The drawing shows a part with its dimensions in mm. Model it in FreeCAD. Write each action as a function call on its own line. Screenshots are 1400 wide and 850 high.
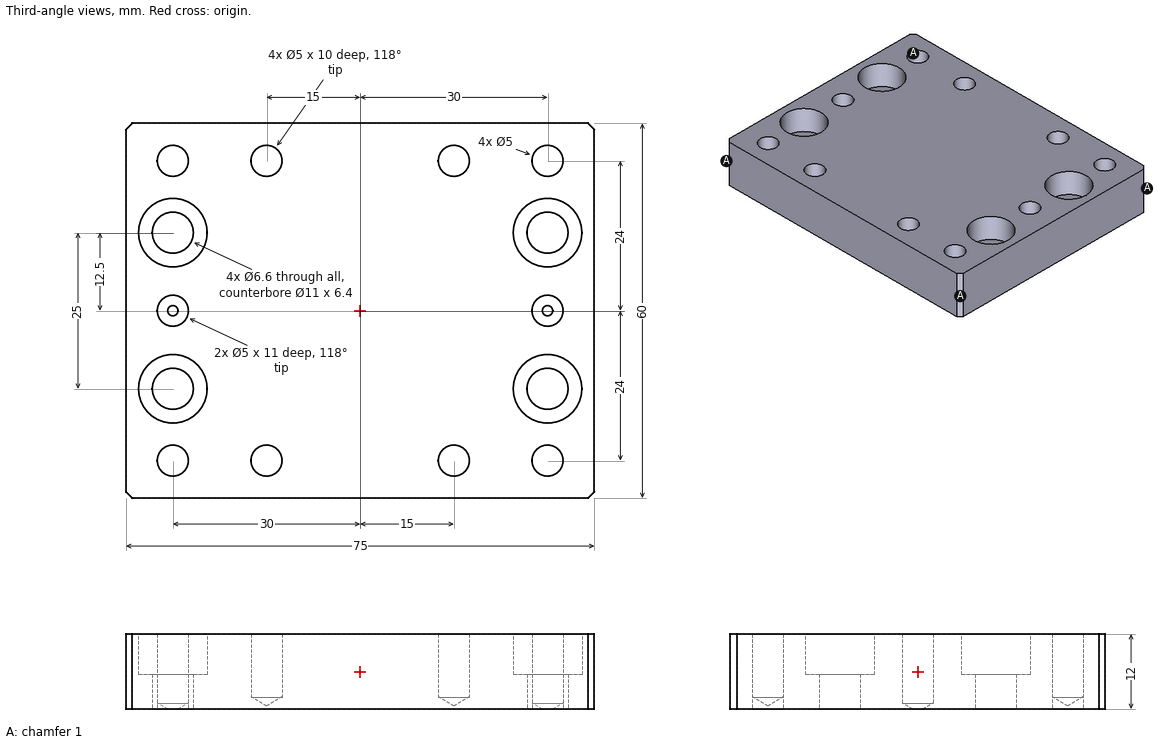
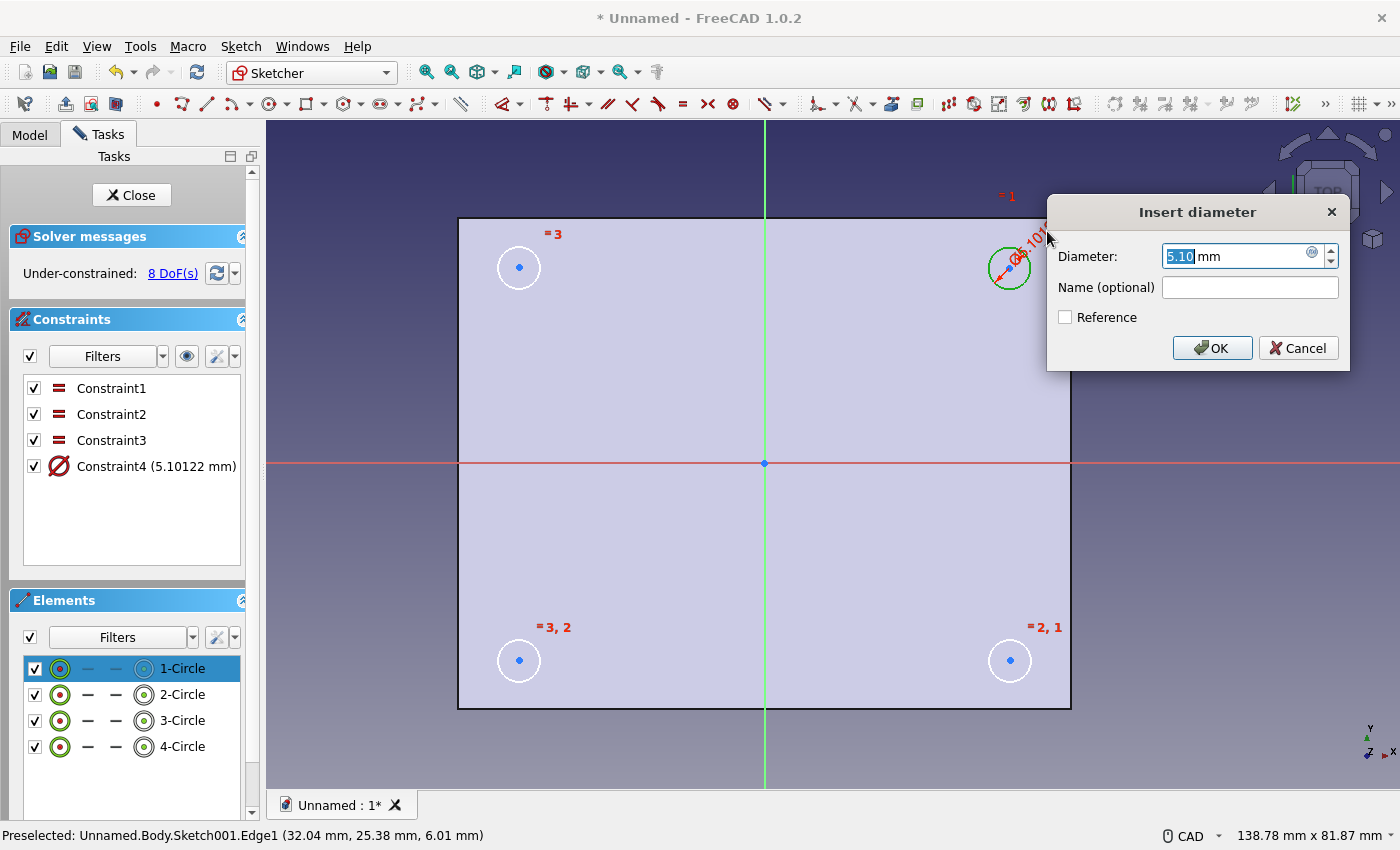
text(5)
key(Return)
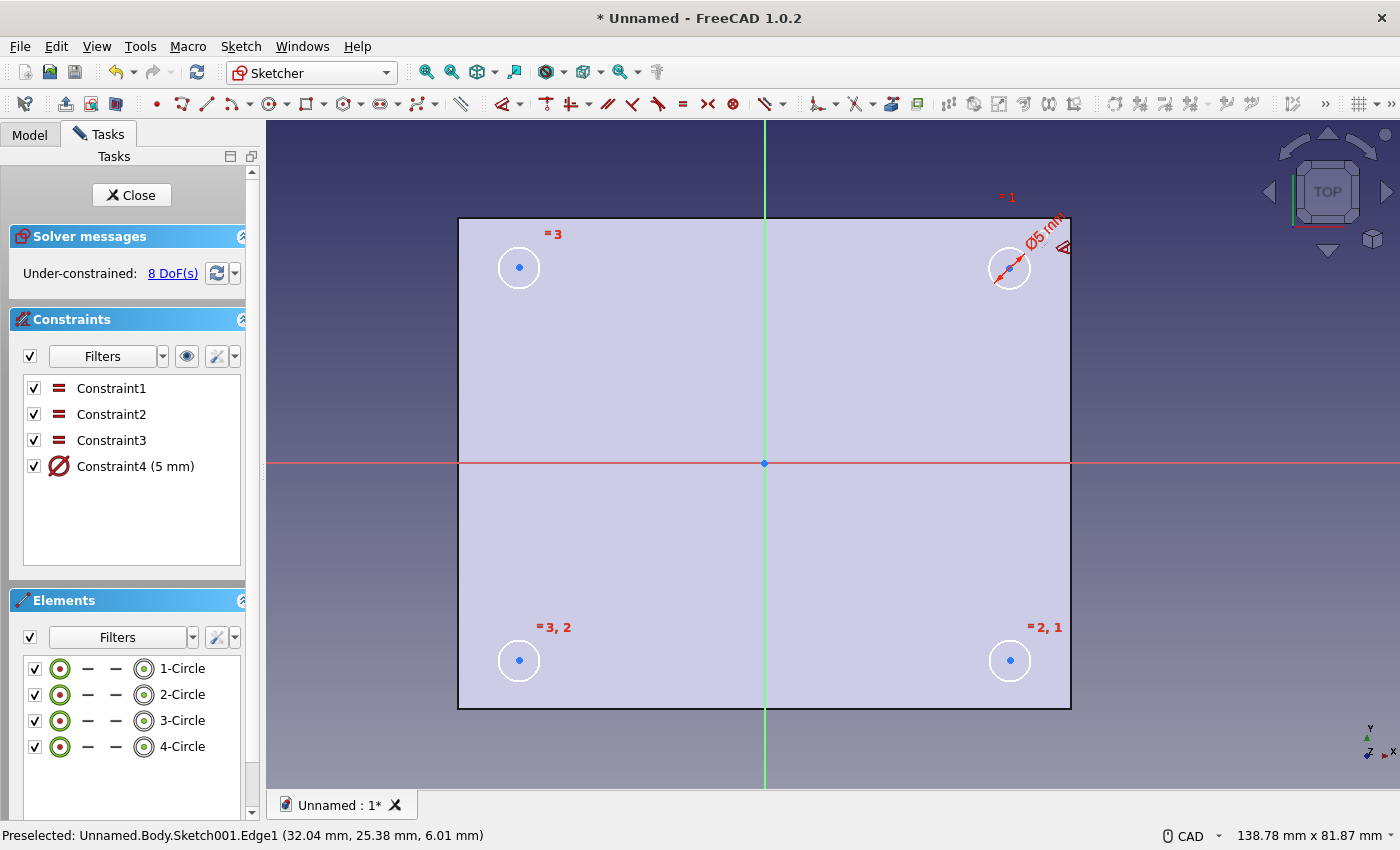
click(1010, 268)
click(887, 234)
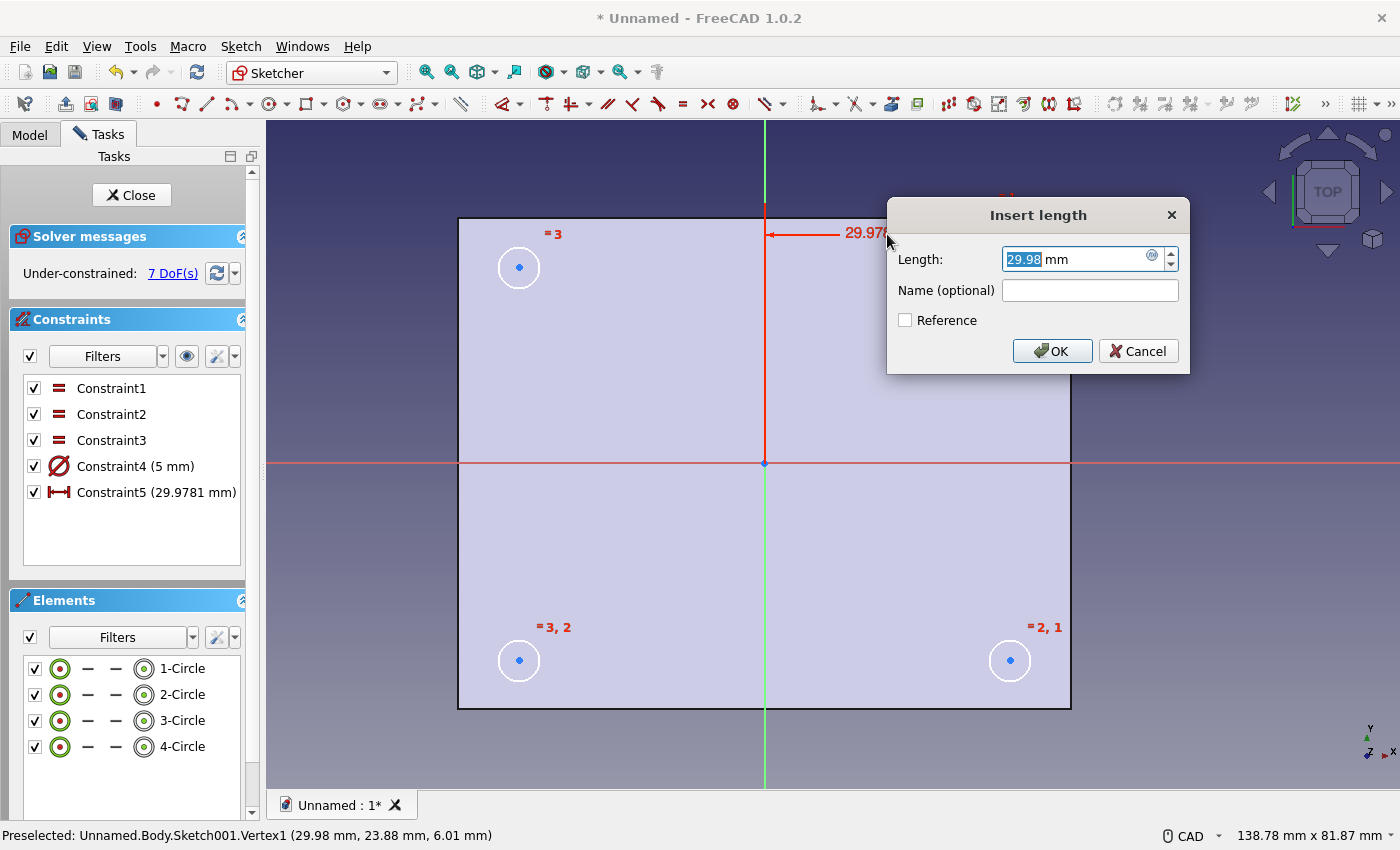
text(30)
key(Return)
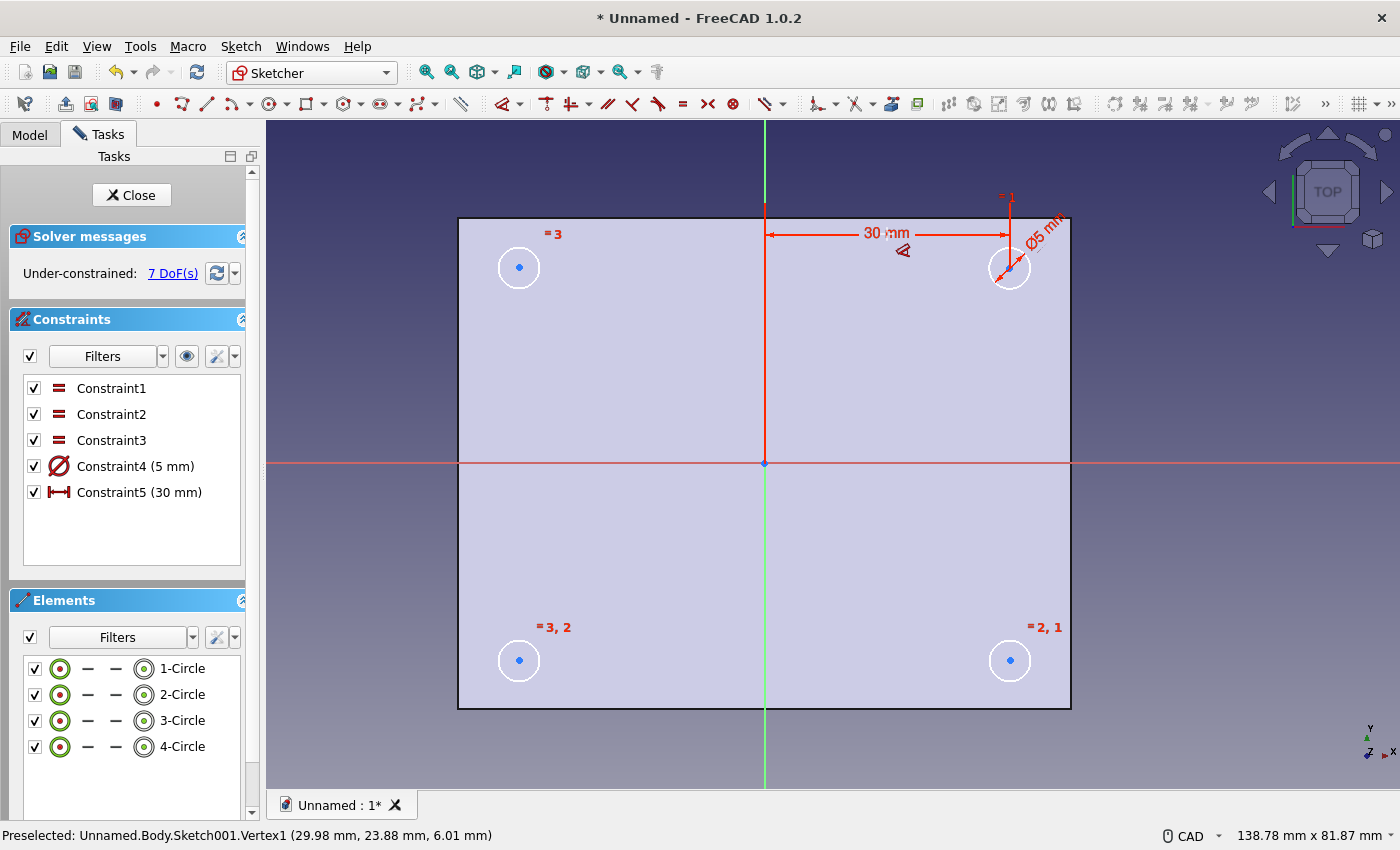
click(1010, 268)
click(1044, 366)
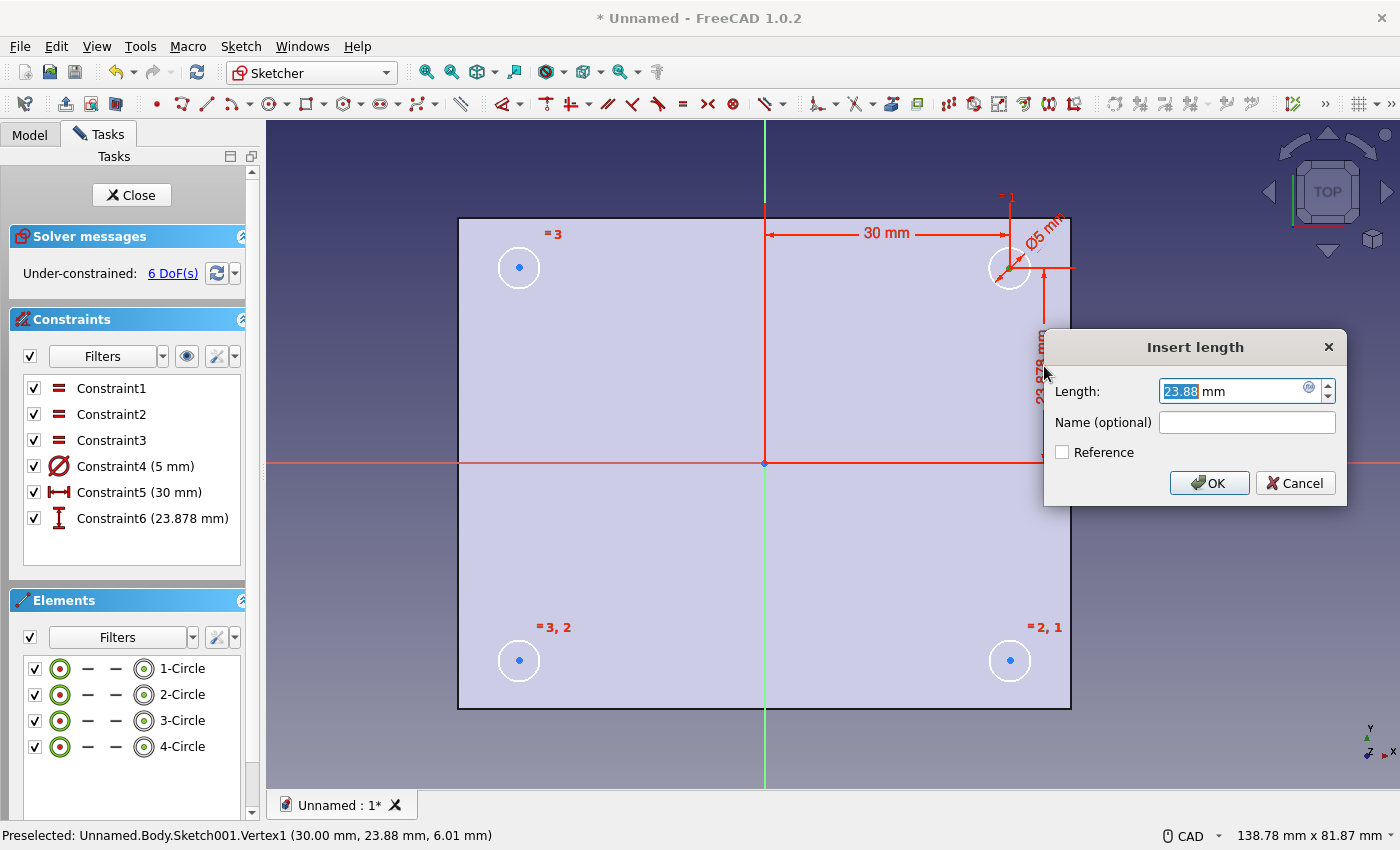
text(24)
key(Return)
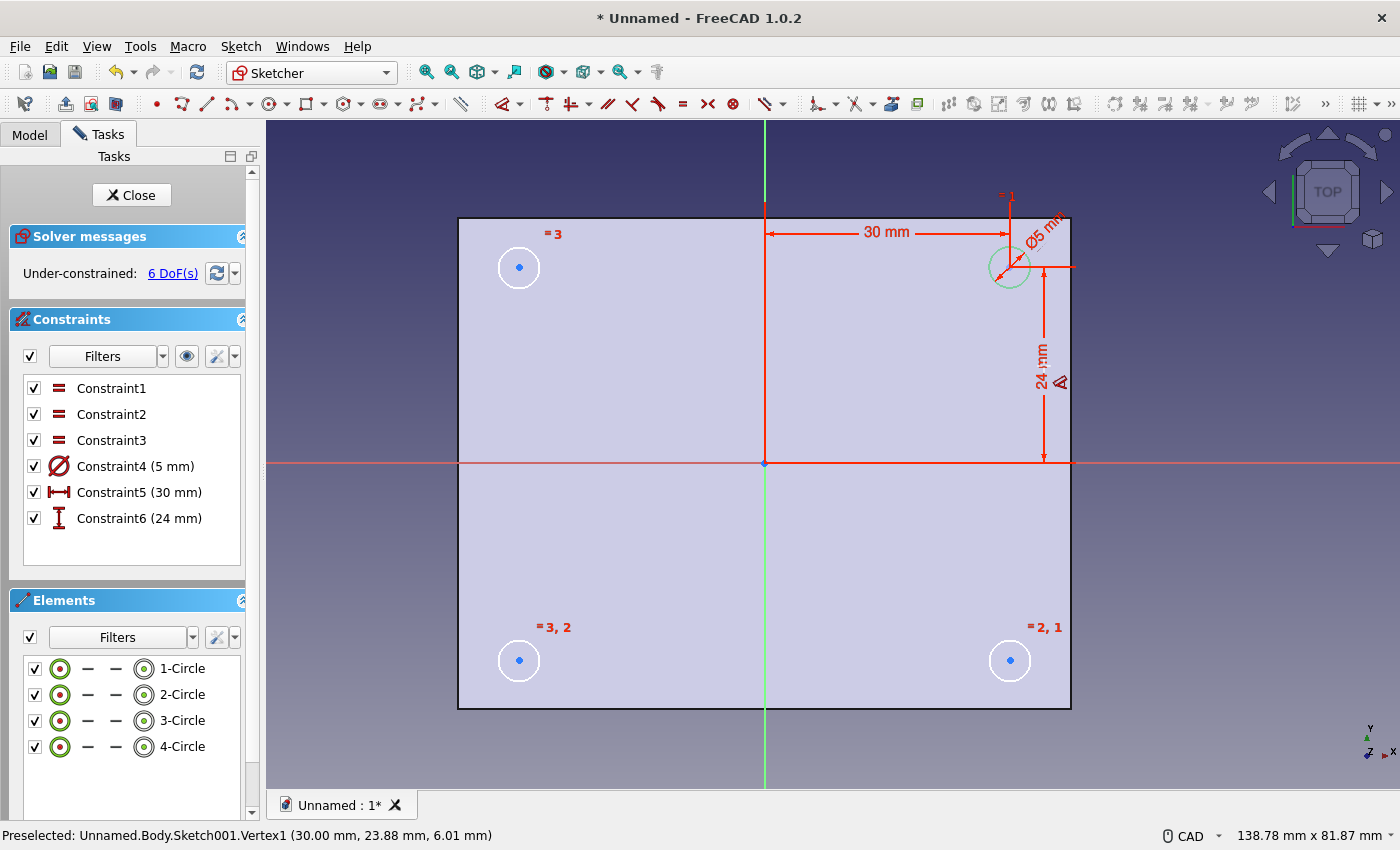
click(1010, 661)
click(887, 695)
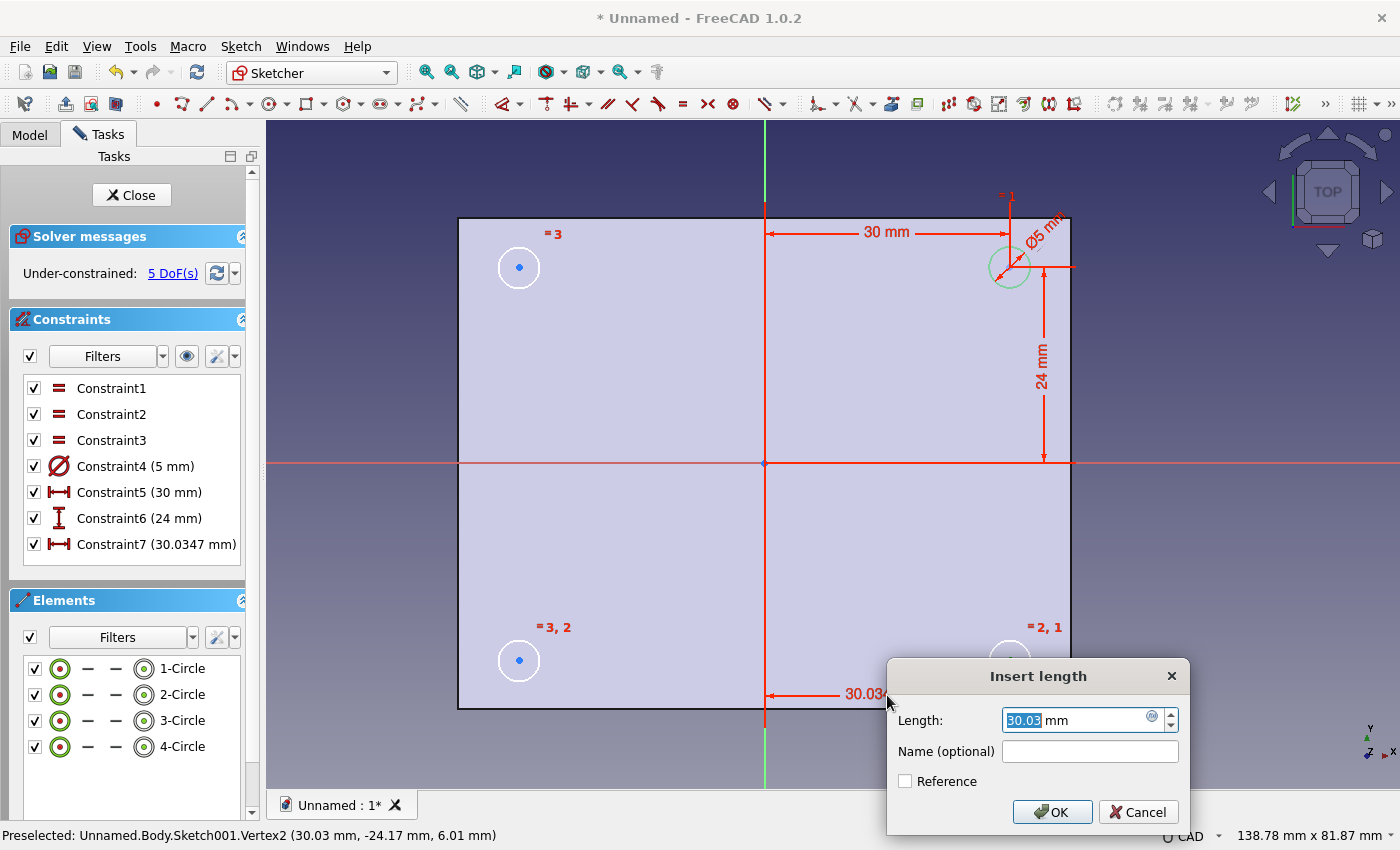
text(30)
key(Return)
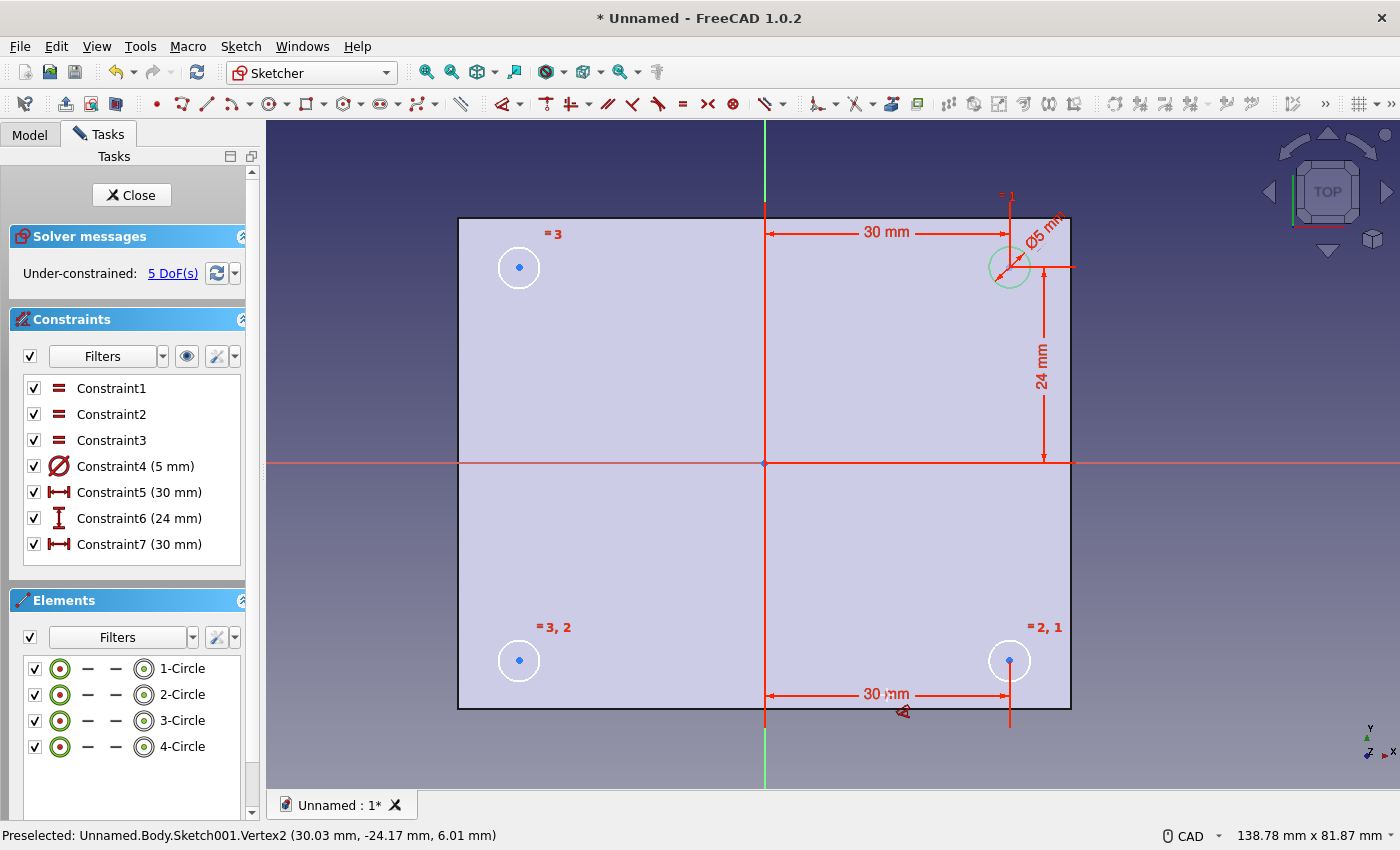
click(1010, 661)
click(1044, 562)